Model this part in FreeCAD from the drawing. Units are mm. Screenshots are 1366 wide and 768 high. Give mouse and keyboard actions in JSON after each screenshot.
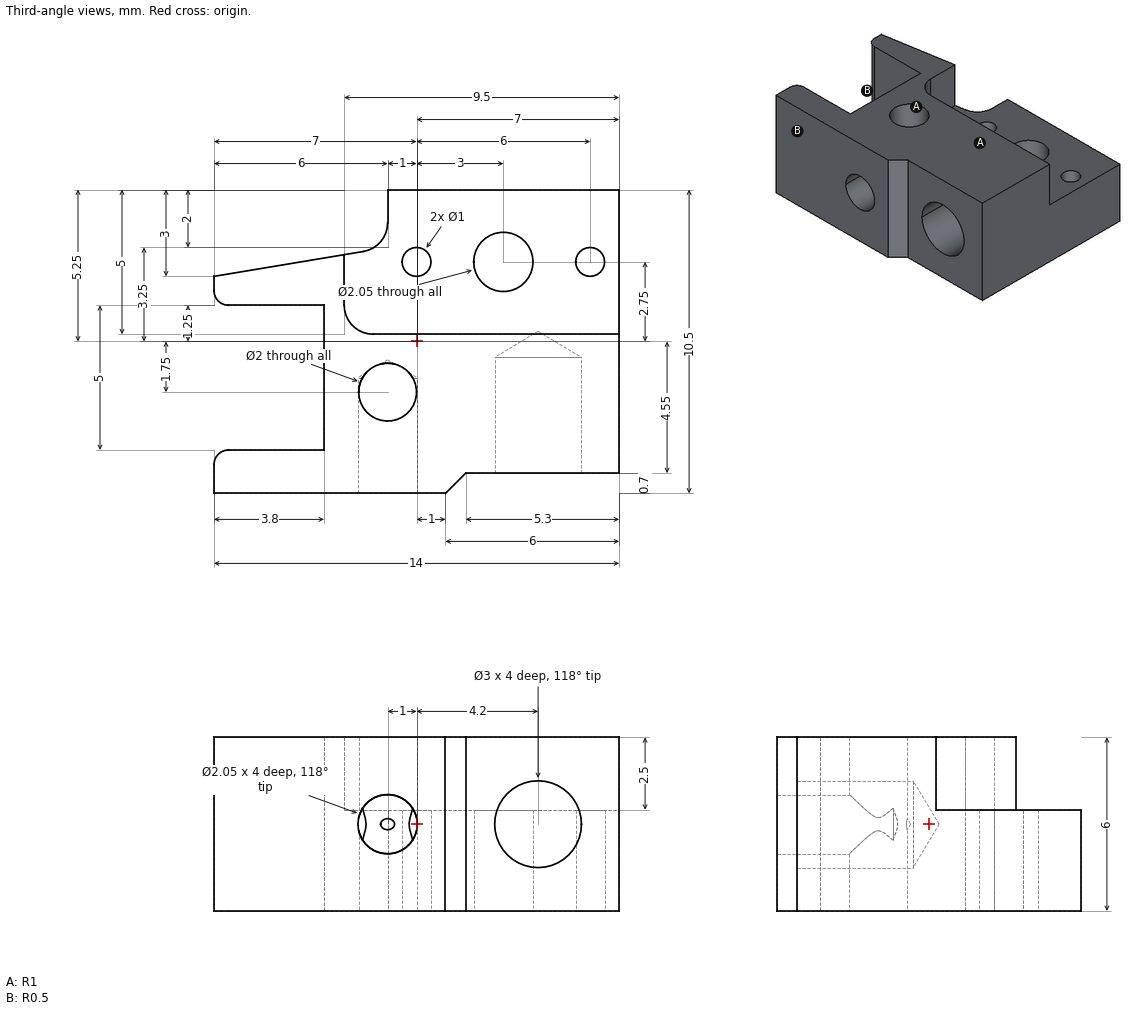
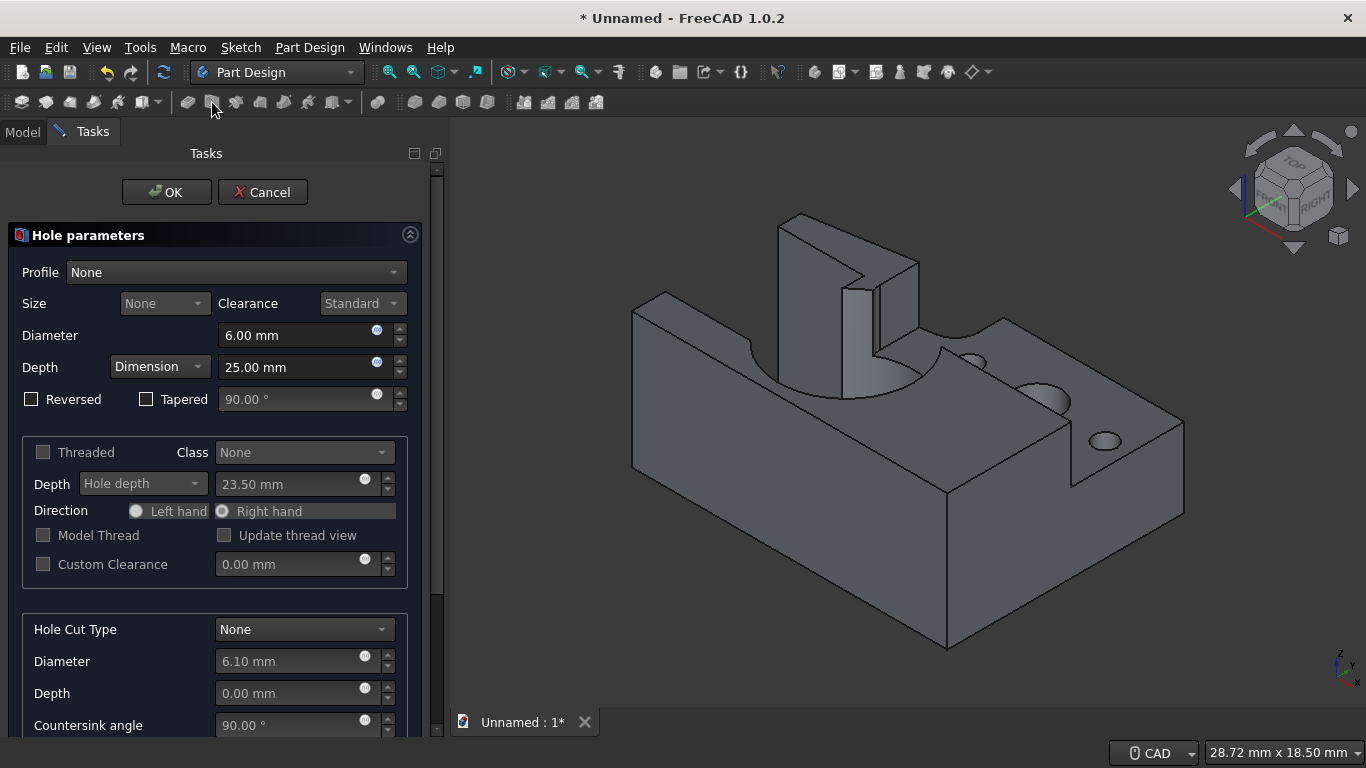
{"action": "triple_click", "coordinate": [305, 335]}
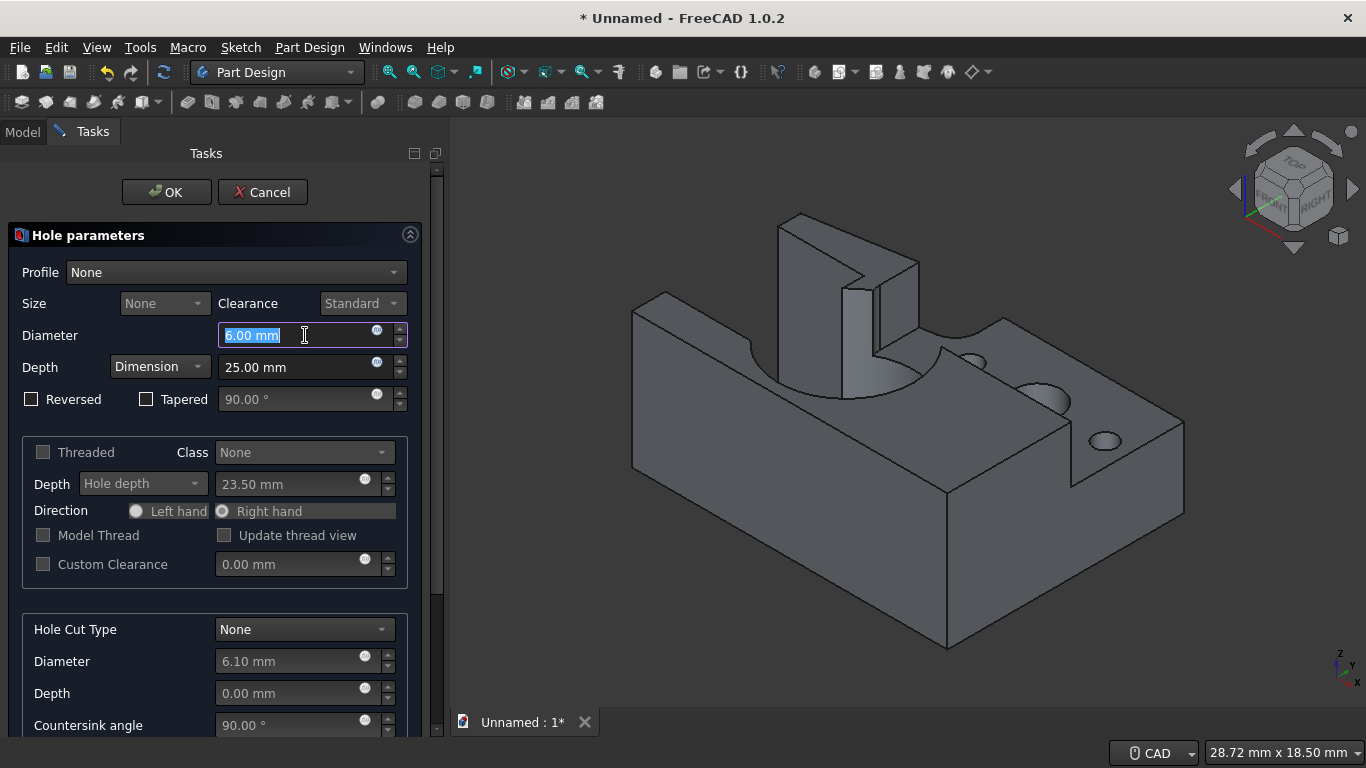
{"action": "type", "text": "2"}
{"action": "key", "text": "Tab"}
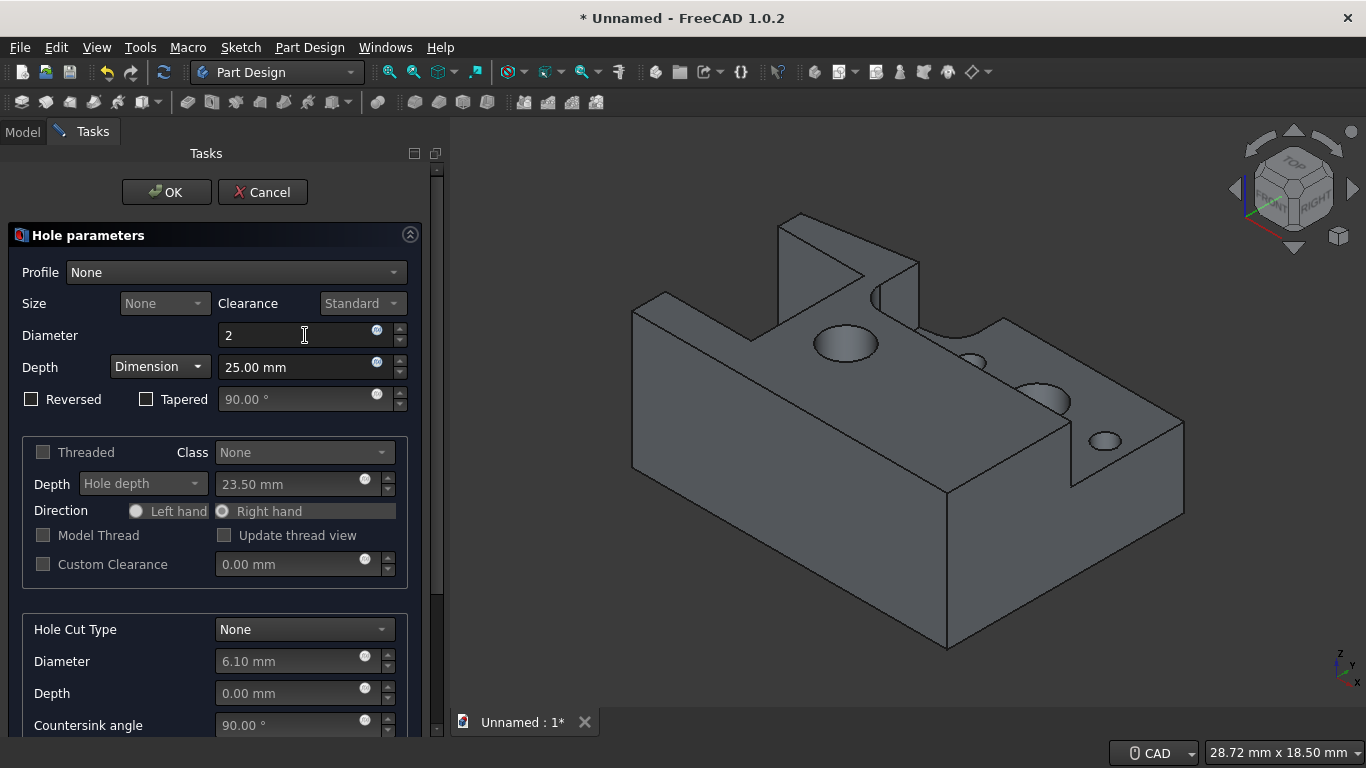
{"action": "left_click", "coordinate": [161, 366]}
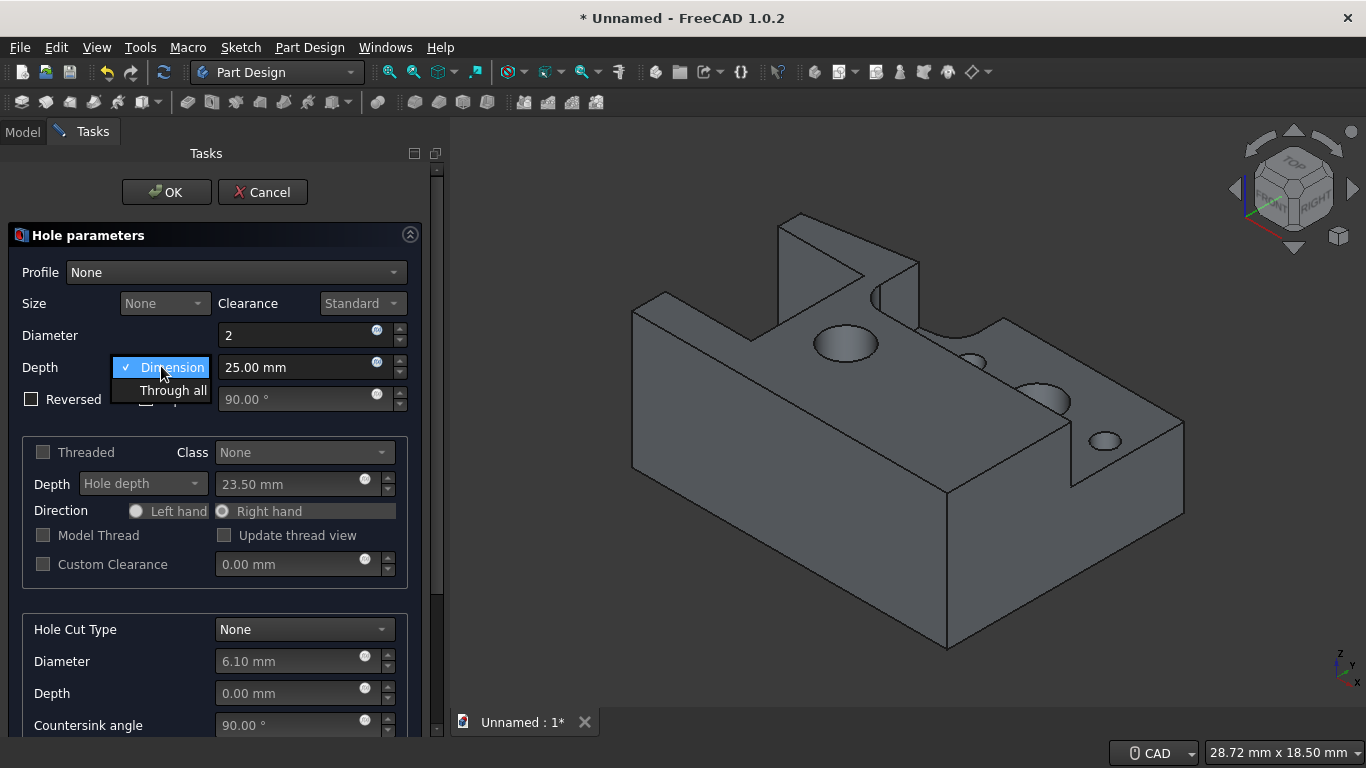
{"action": "left_click", "coordinate": [160, 390]}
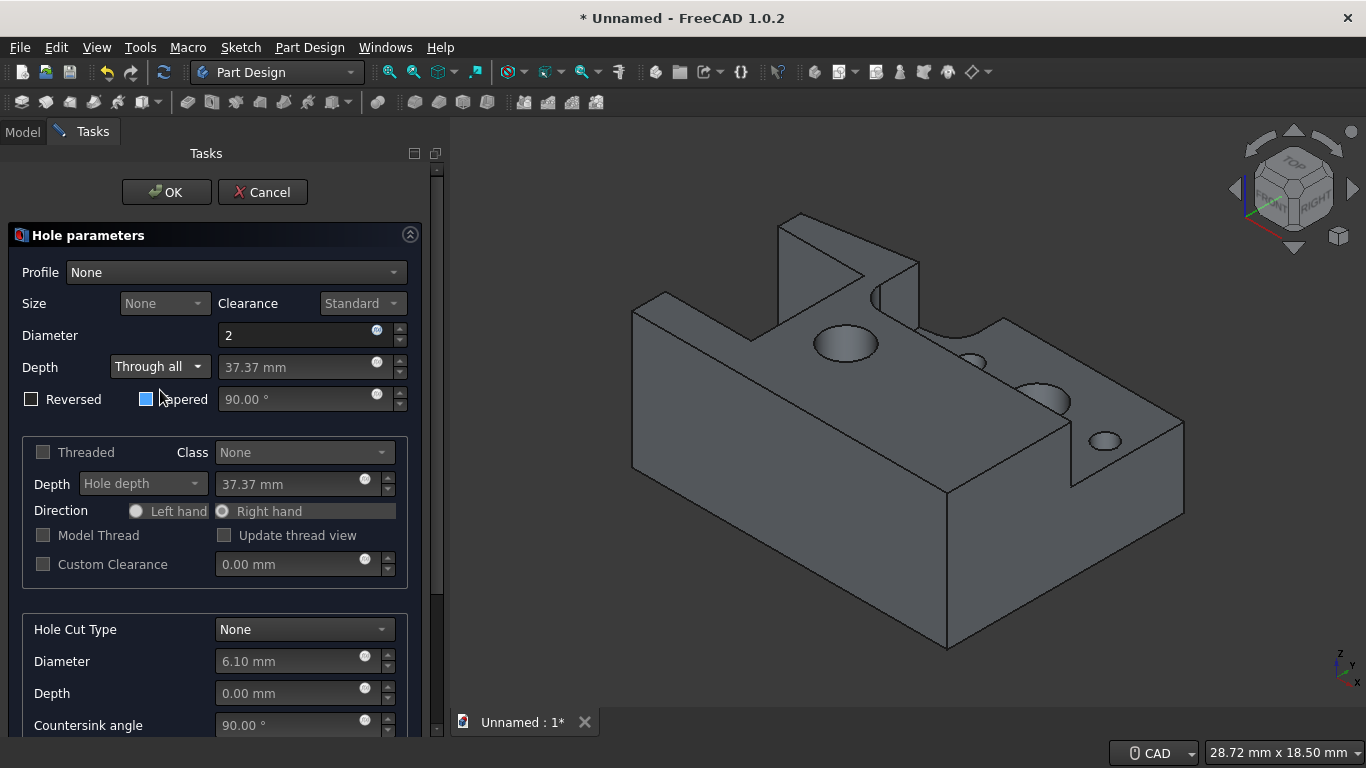
{"action": "left_click", "coordinate": [167, 192]}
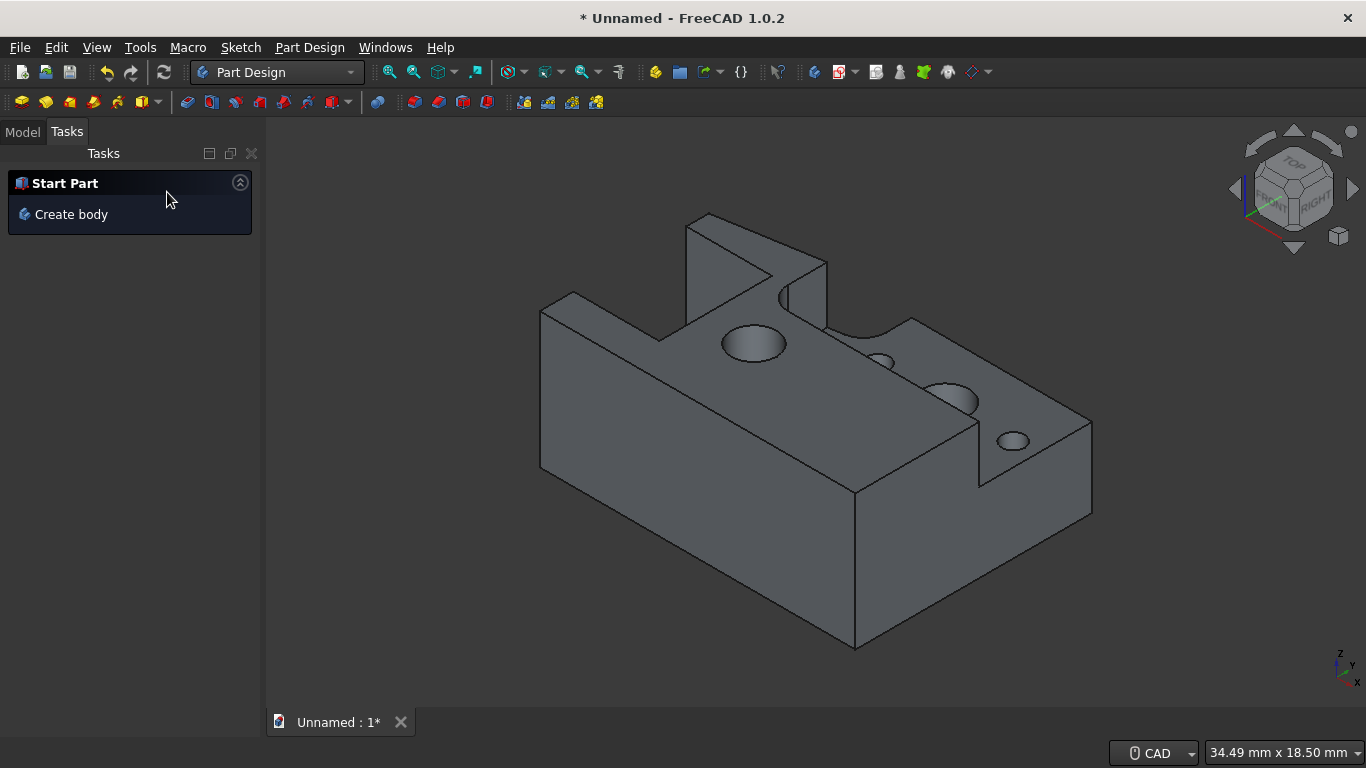
{"action": "left_click", "coordinate": [854, 415]}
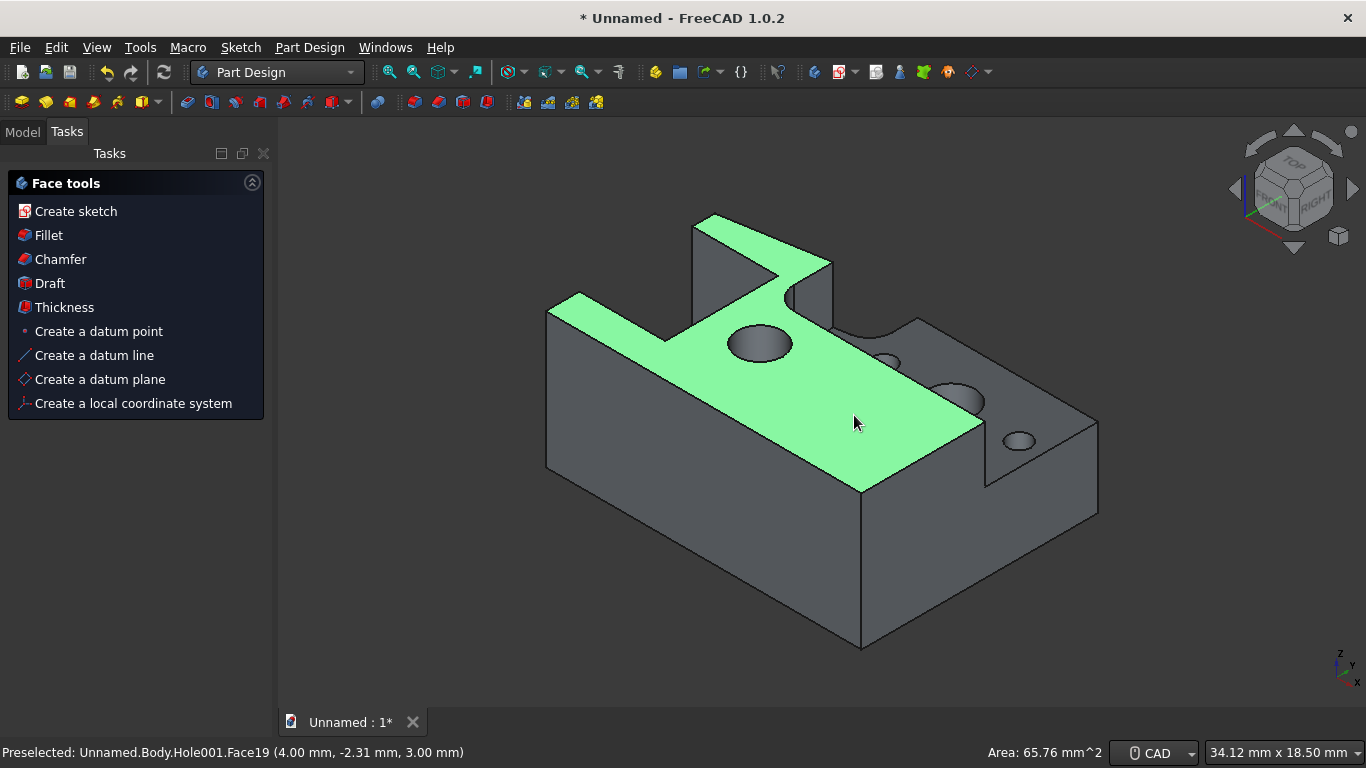
{"action": "left_click", "coordinate": [840, 72]}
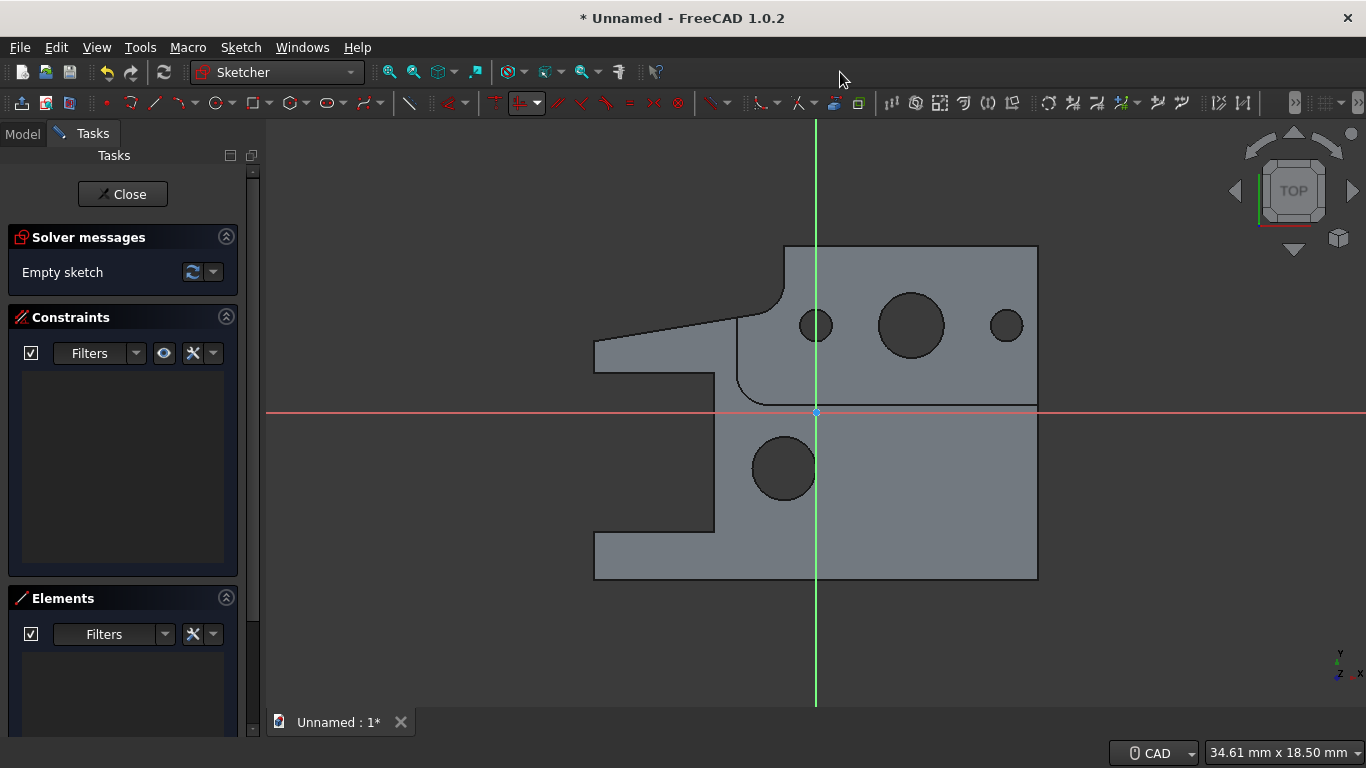
{"action": "scroll", "coordinate": [1074, 565], "scroll_direction": "up", "scroll_amount": 4}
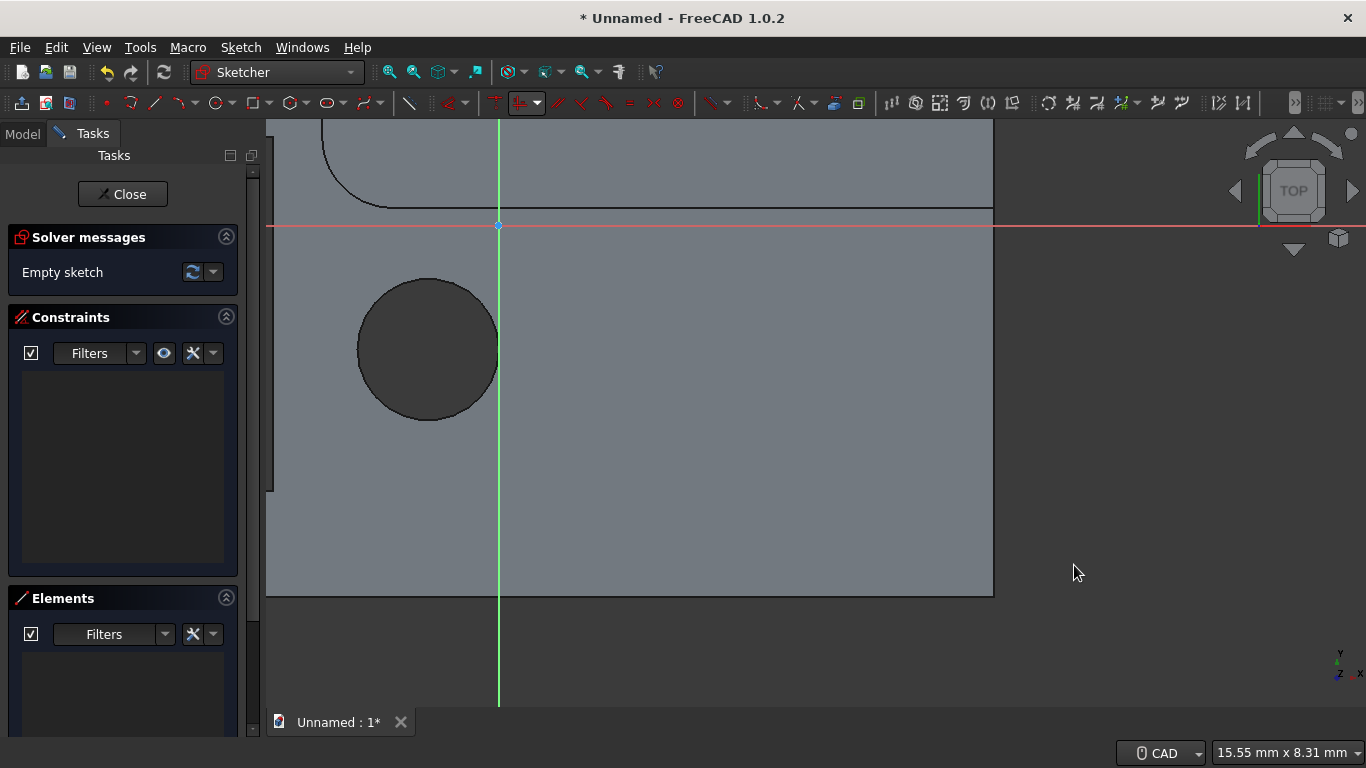
{"action": "left_click", "coordinate": [132, 104]}